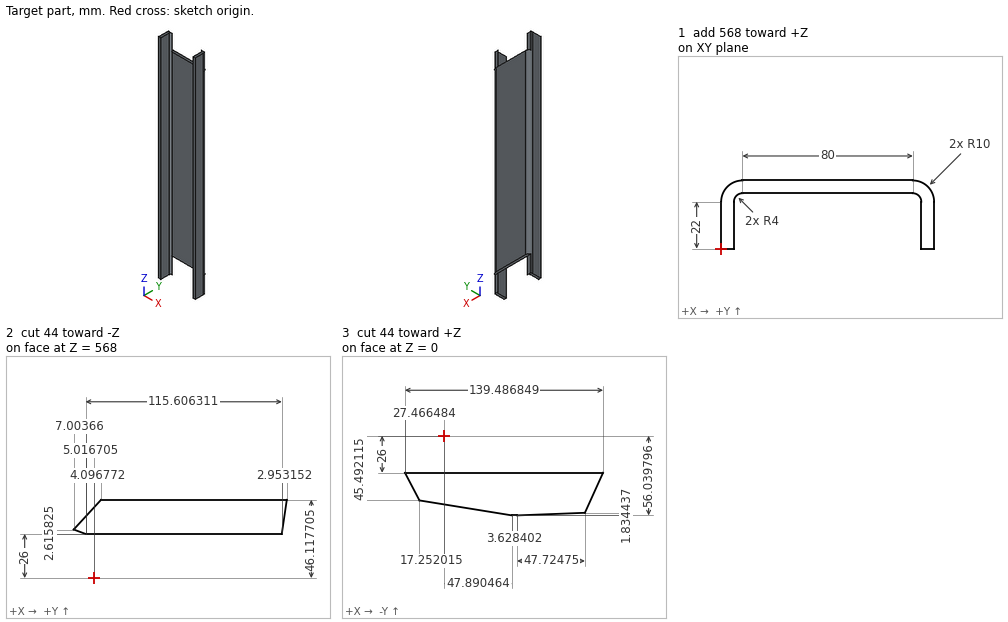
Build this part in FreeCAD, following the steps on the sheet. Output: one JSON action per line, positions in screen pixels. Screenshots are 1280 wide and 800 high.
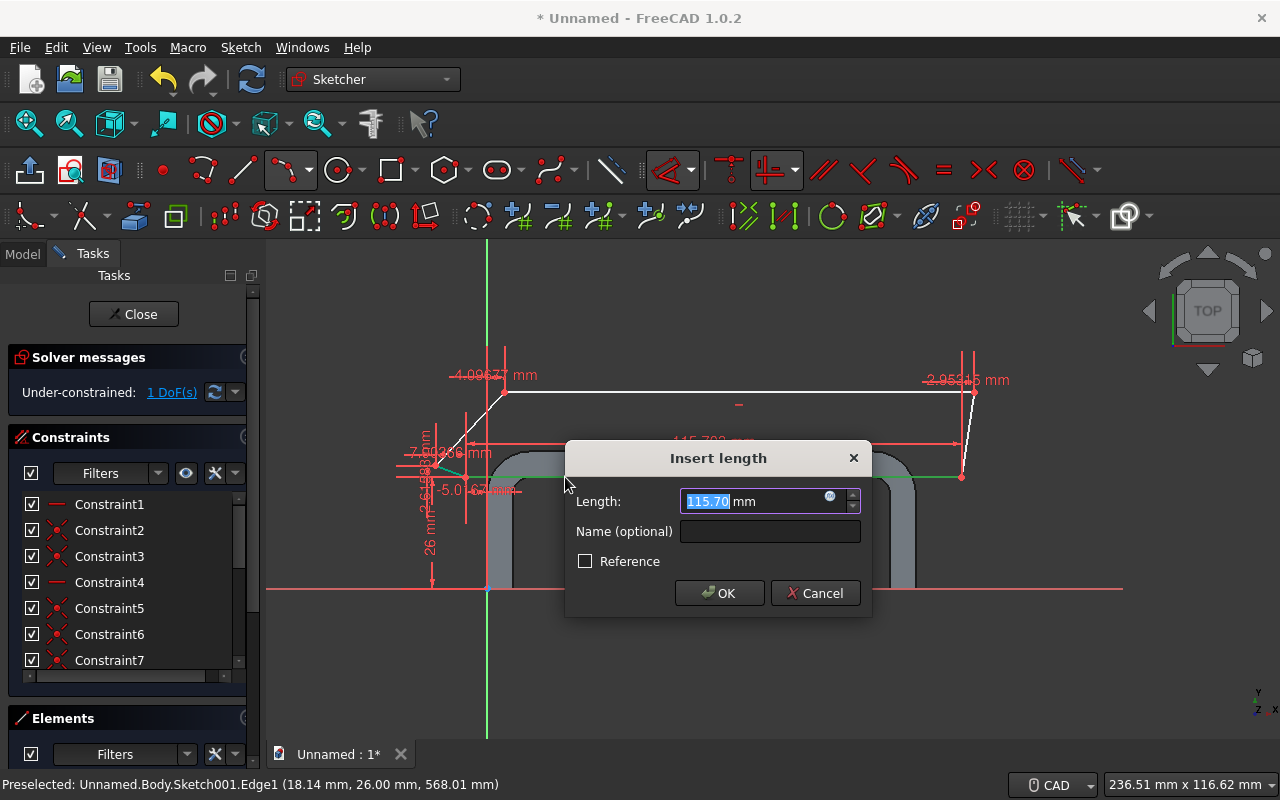
{"action": "type", "text": "115.606311"}
{"action": "key", "text": "Return"}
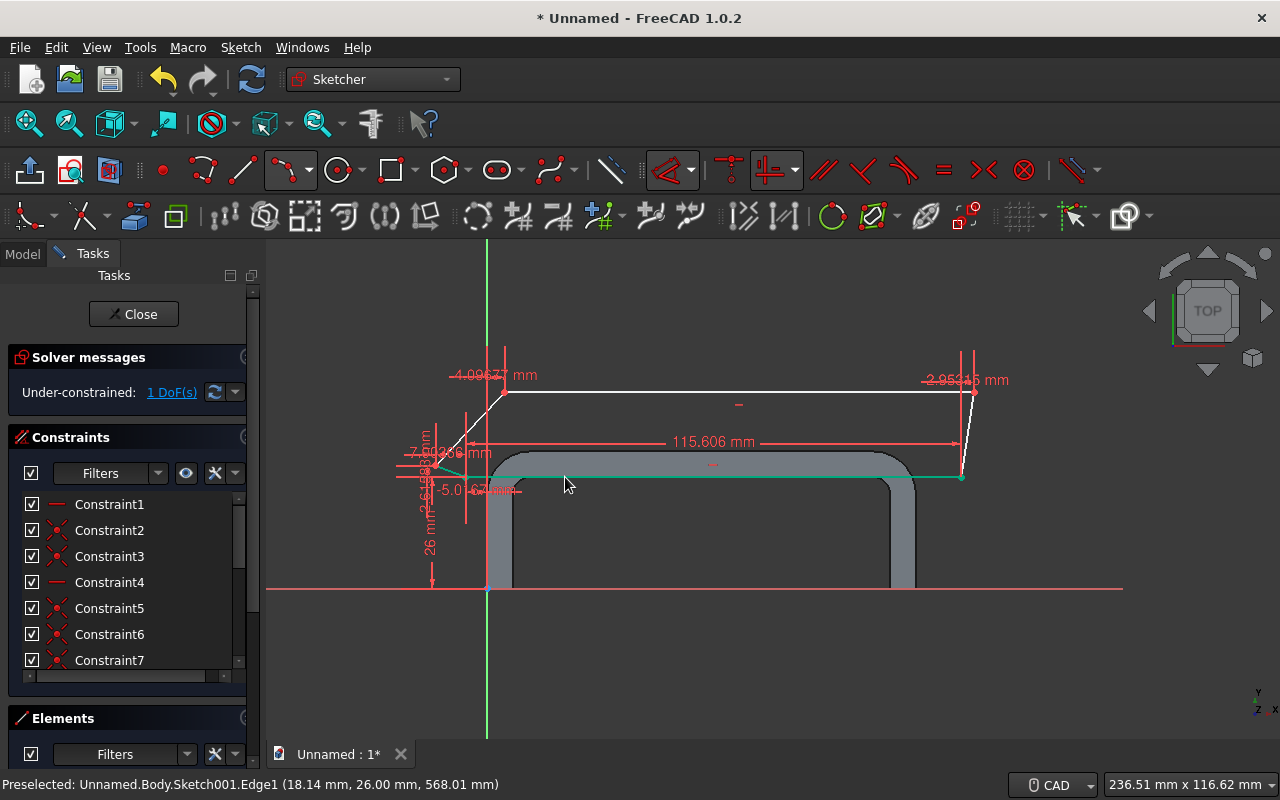
{"action": "left_click", "coordinate": [974, 392]}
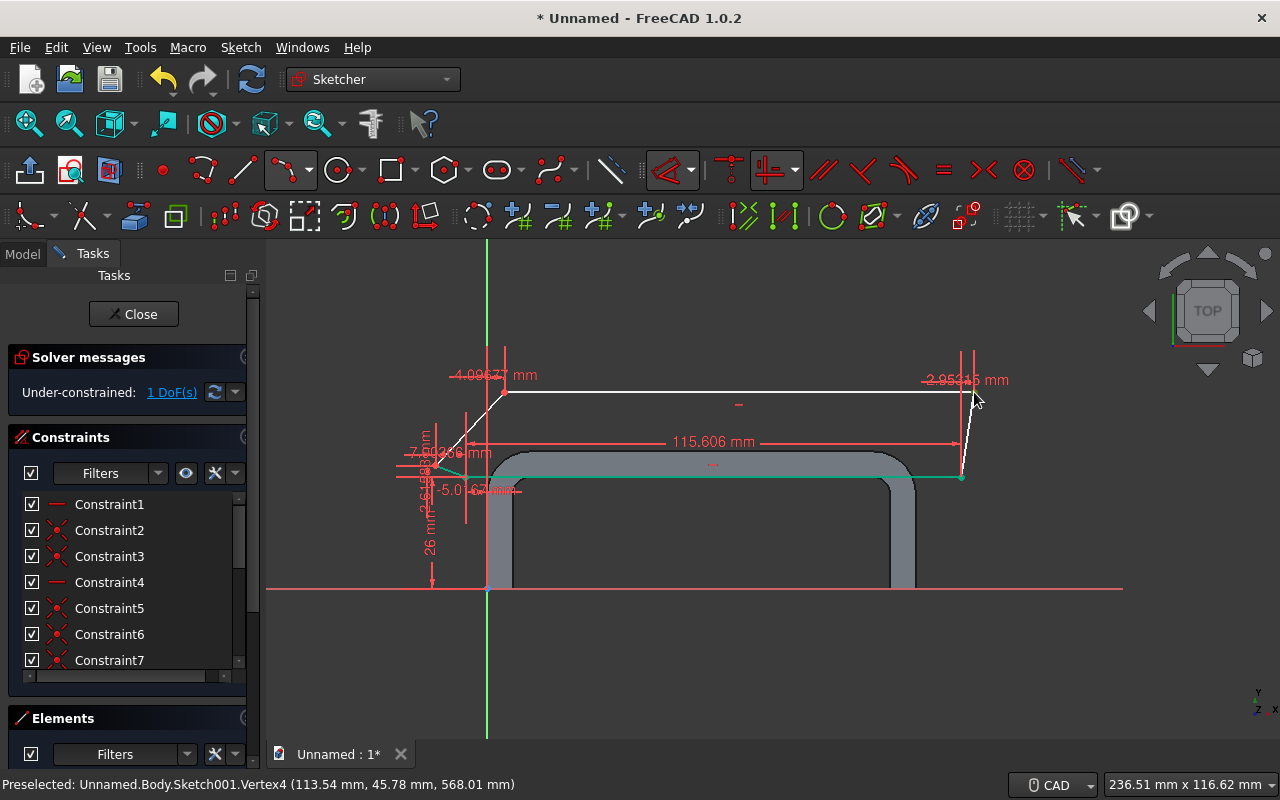
{"action": "left_click", "coordinate": [694, 170]}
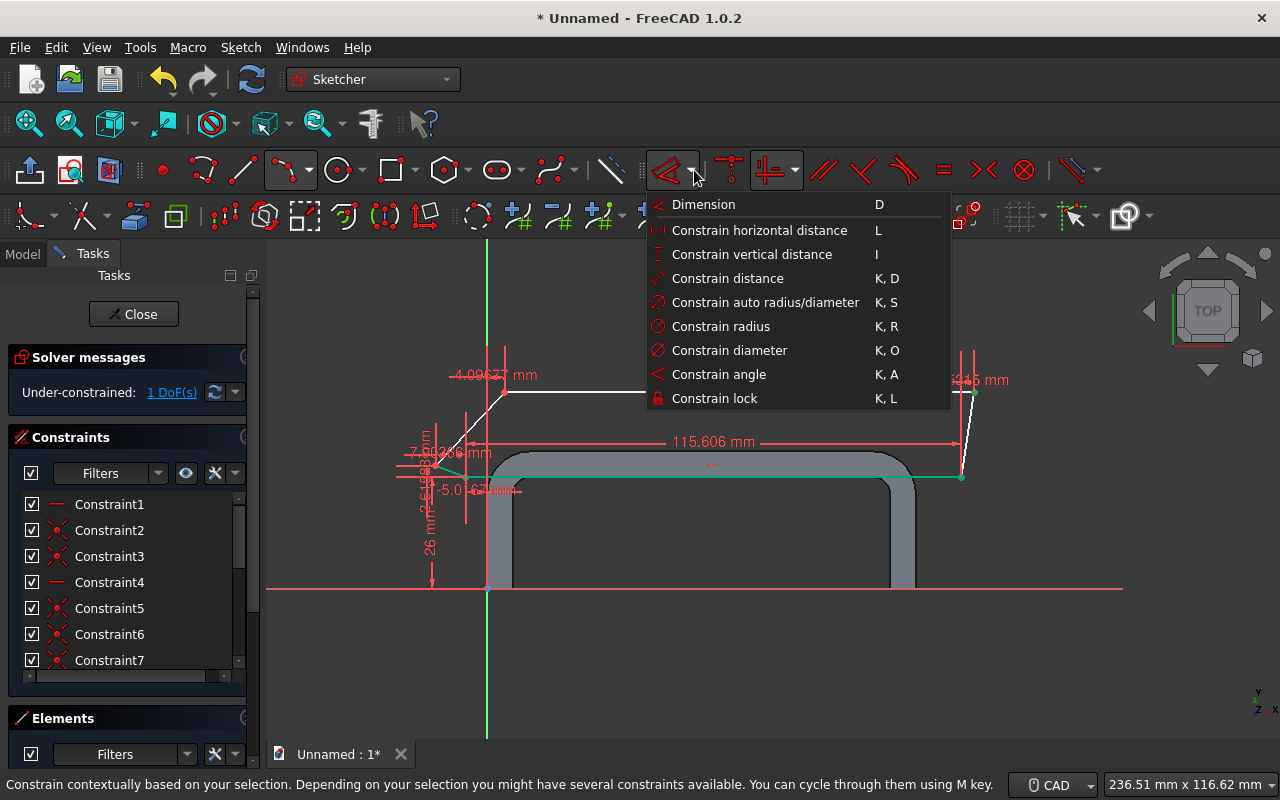
{"action": "left_click", "coordinate": [799, 254]}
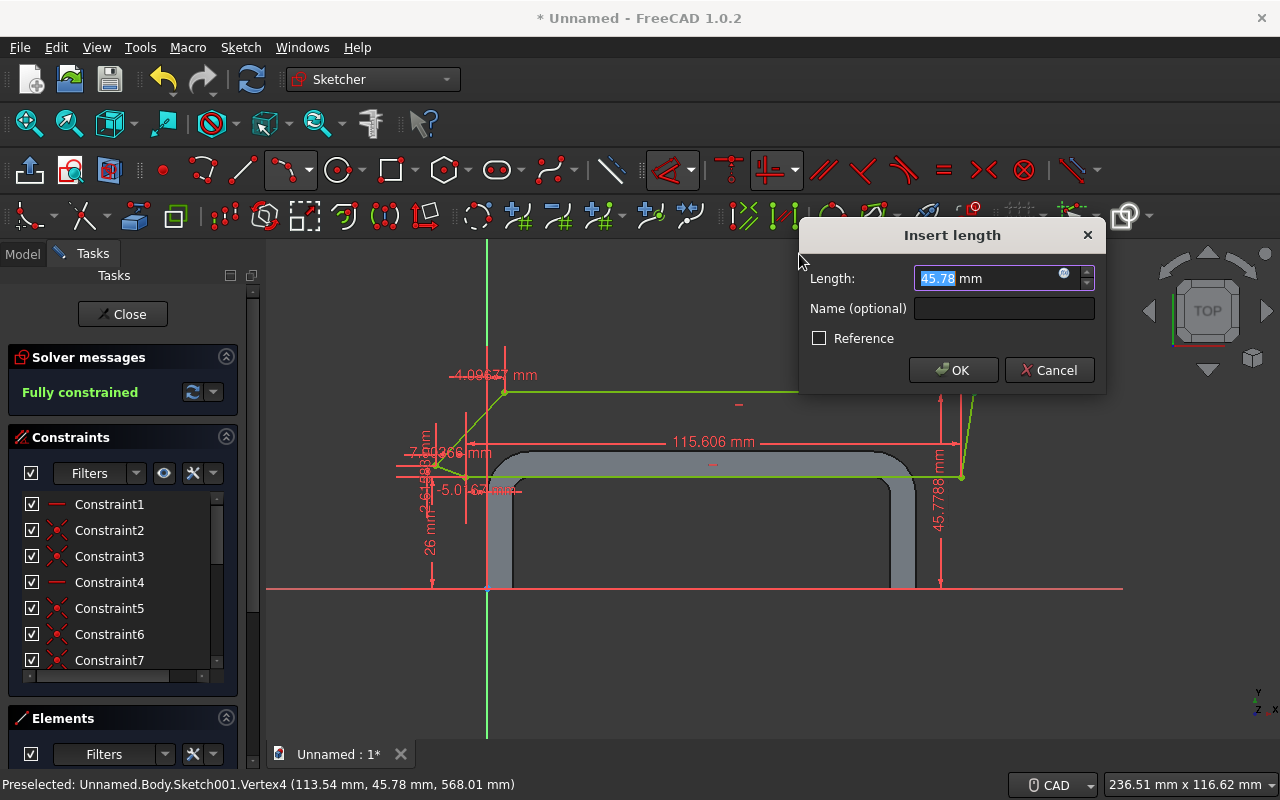
{"action": "type", "text": "46.117705"}
{"action": "key", "text": "Return"}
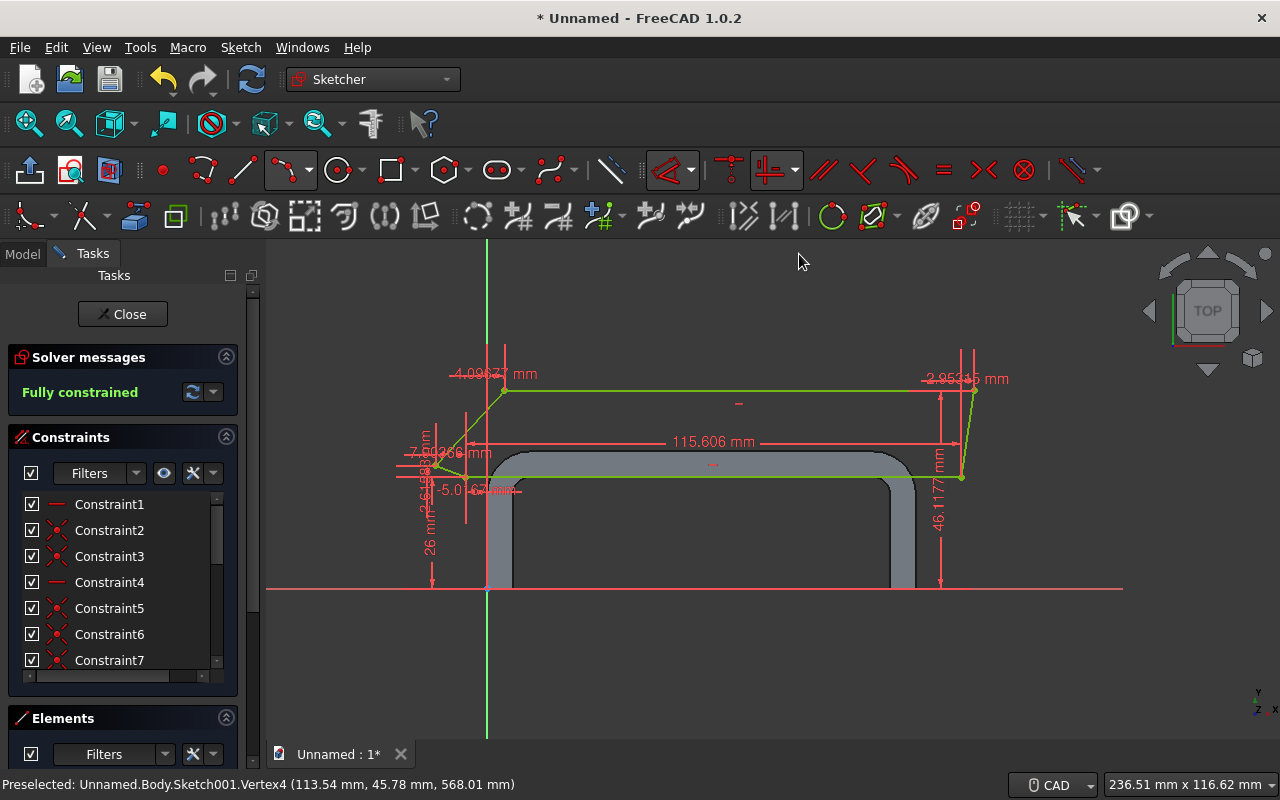
{"action": "left_click", "coordinate": [123, 314]}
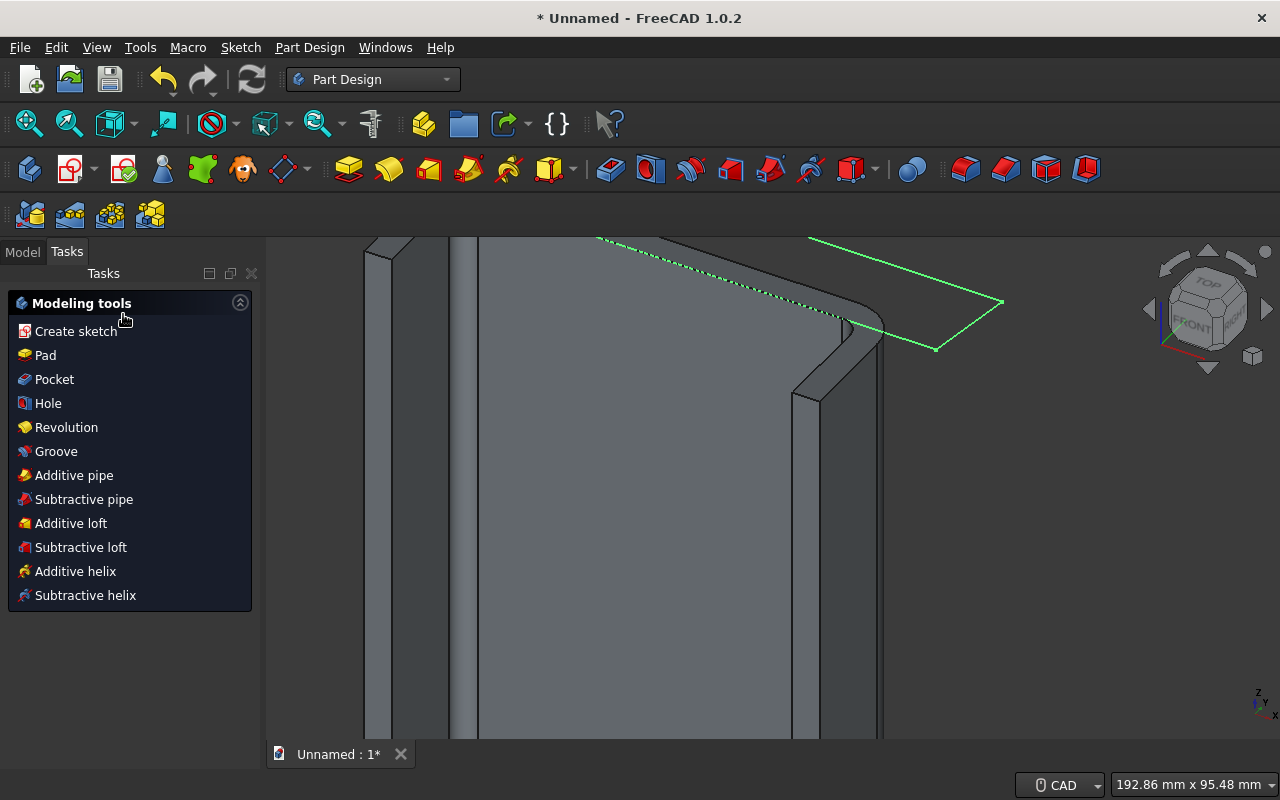
{"action": "left_click", "coordinate": [612, 170]}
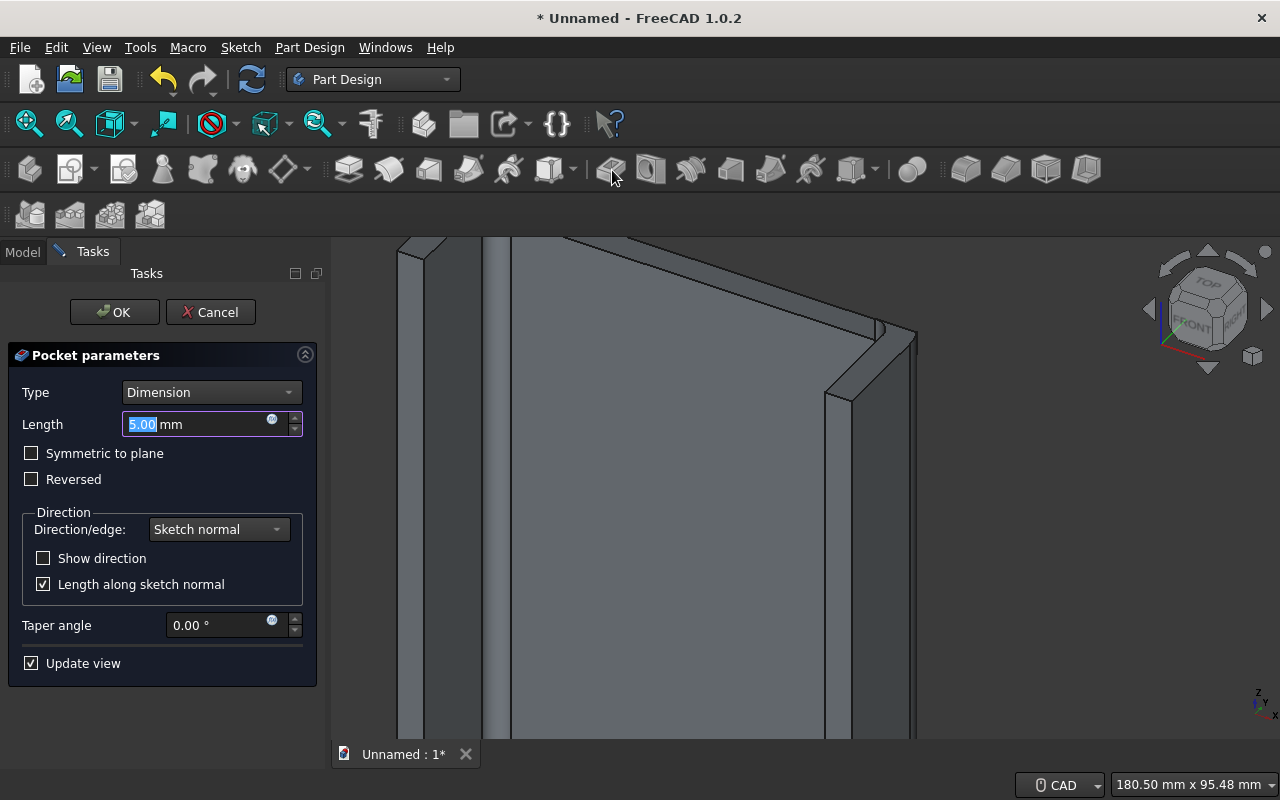
{"action": "type", "text": "44"}
{"action": "key", "text": "Tab"}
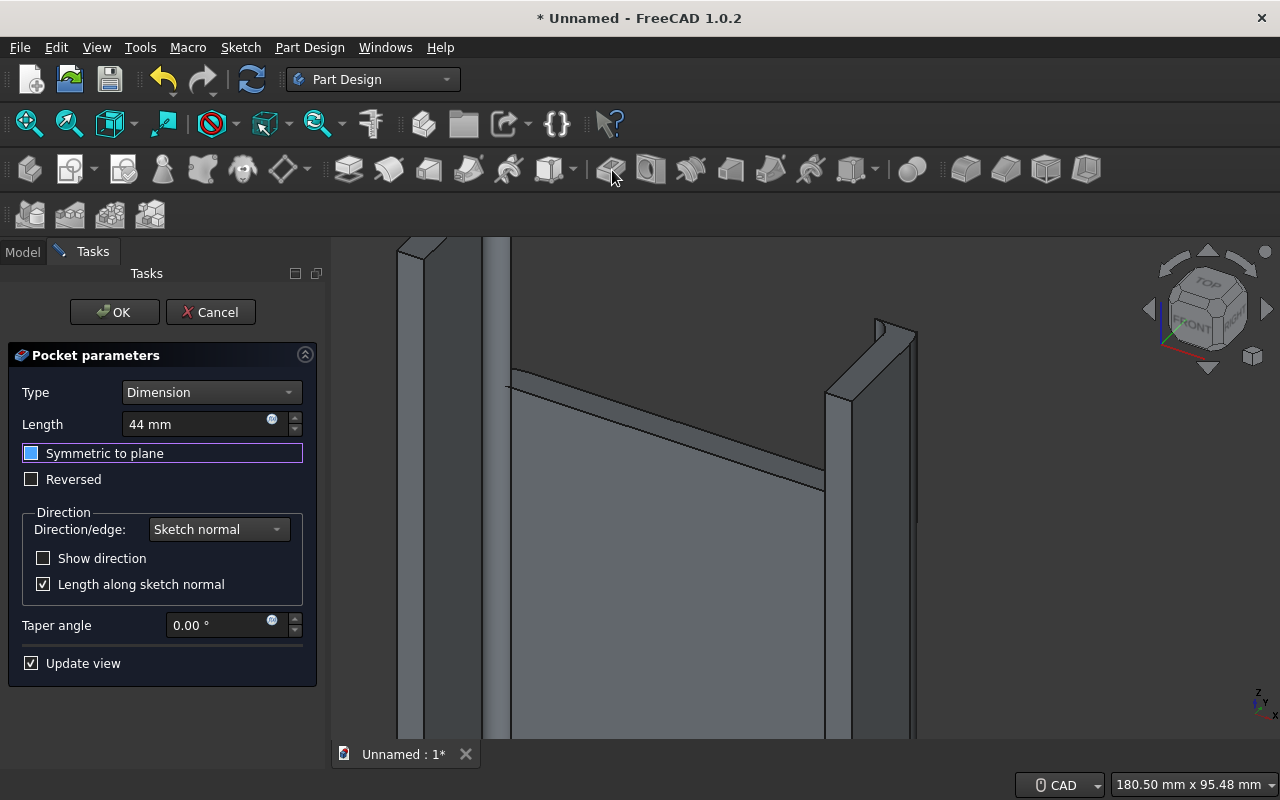
{"action": "left_click", "coordinate": [115, 312]}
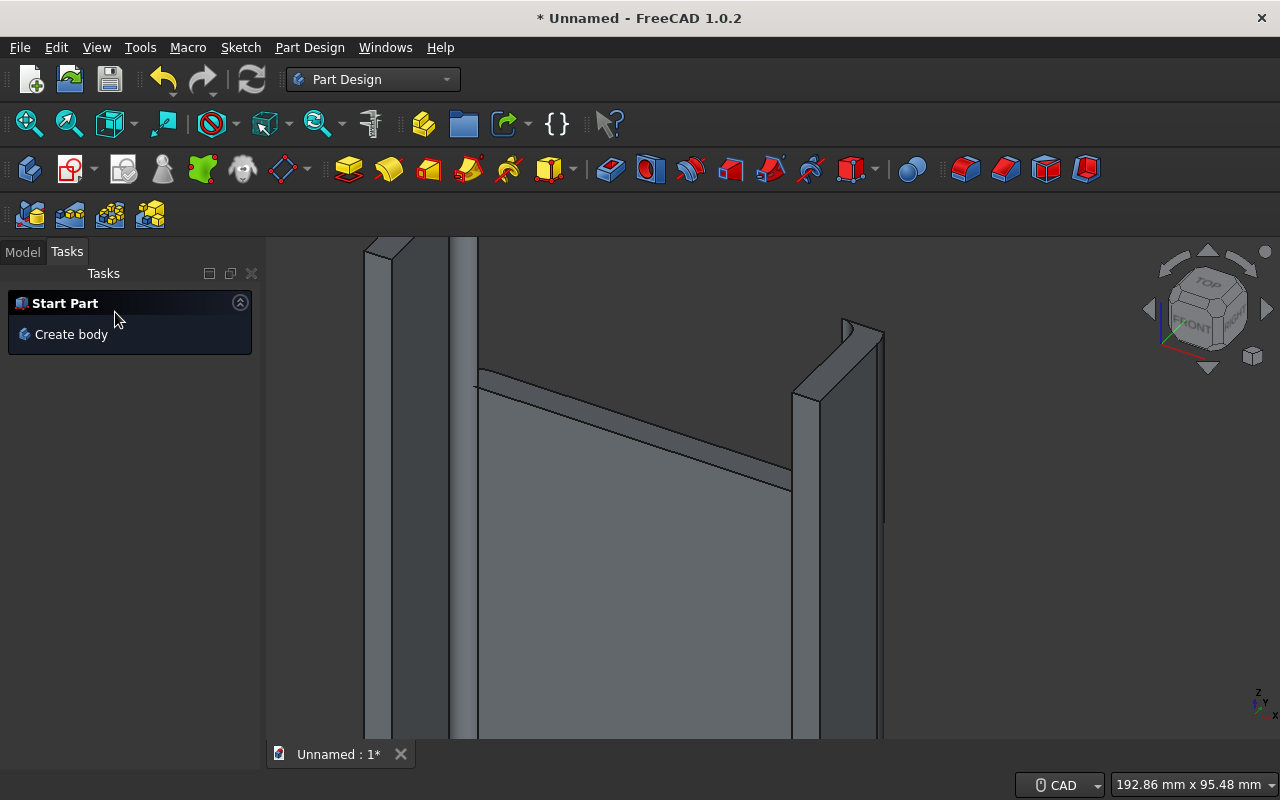
{"action": "left_click", "coordinate": [30, 124]}